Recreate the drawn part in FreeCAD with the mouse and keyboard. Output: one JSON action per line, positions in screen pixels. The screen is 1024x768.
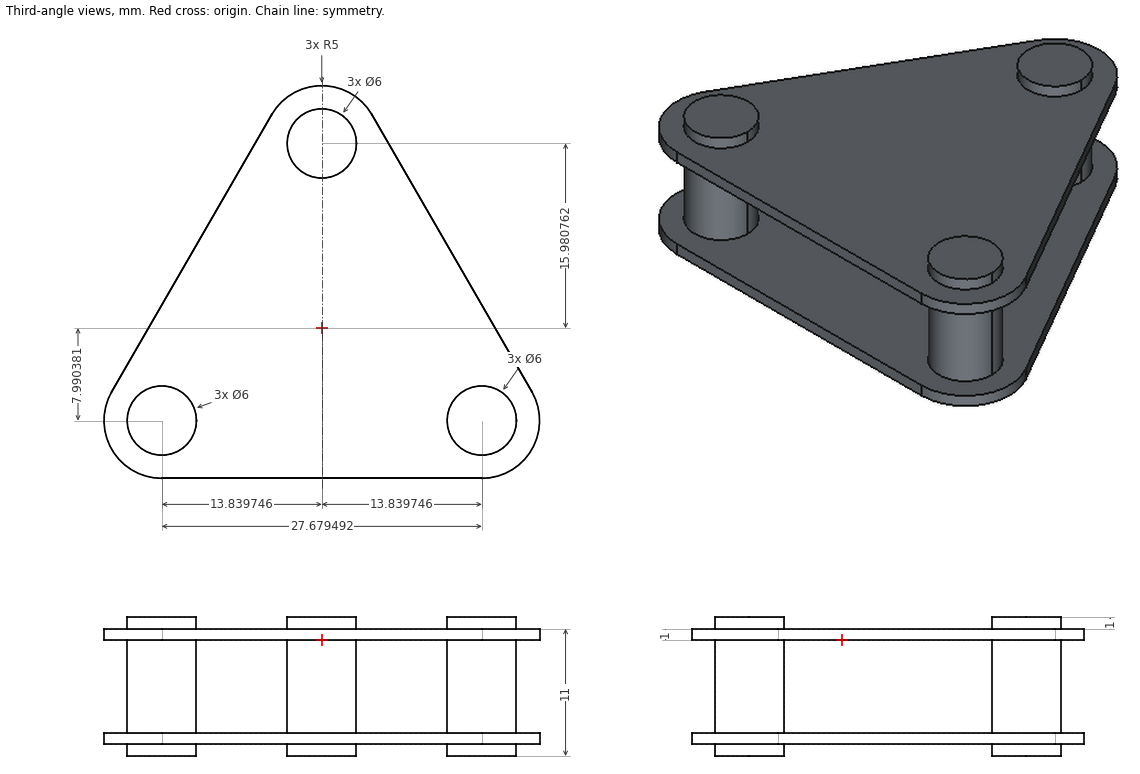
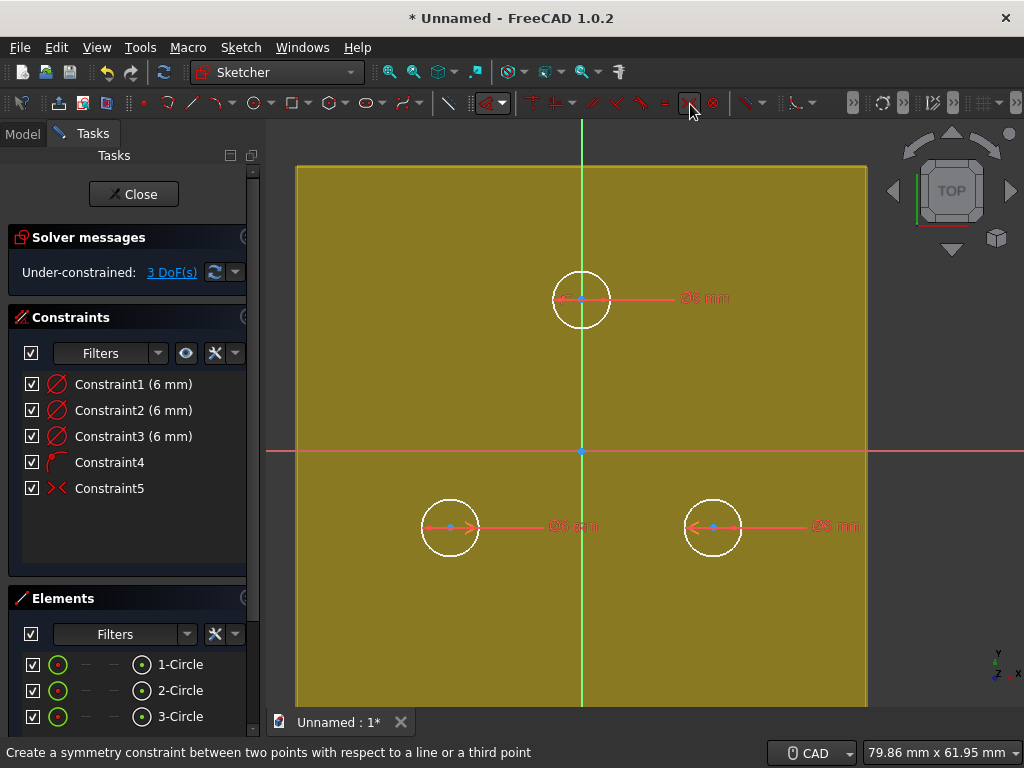
{"action": "left_click", "coordinate": [713, 528]}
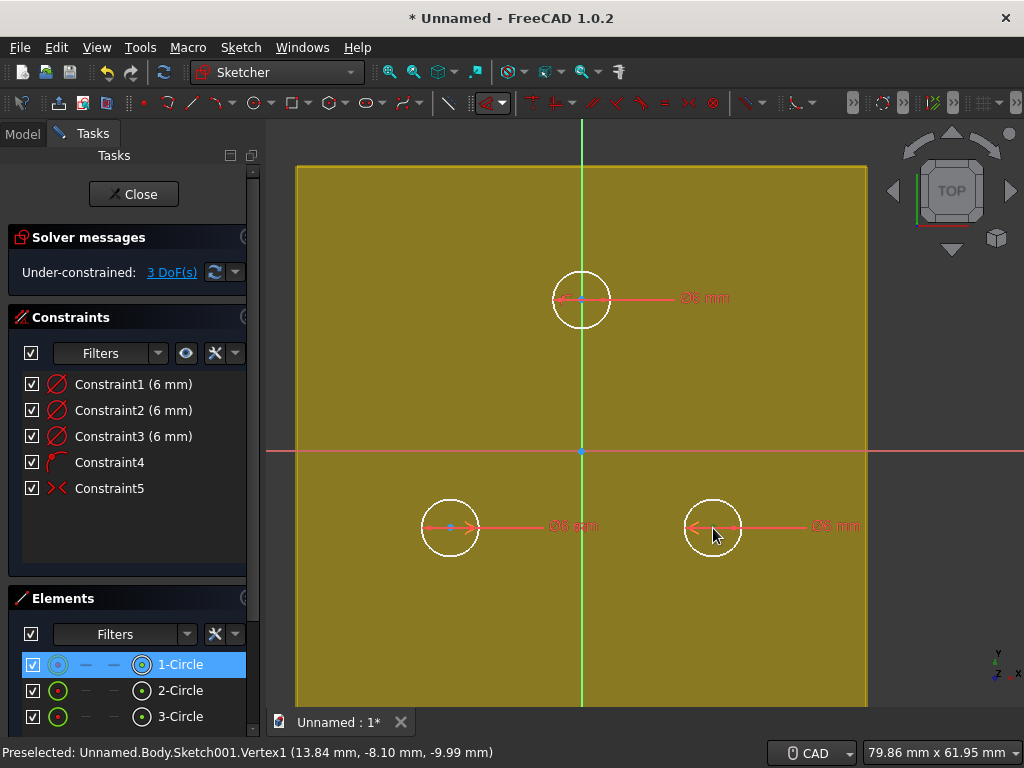
{"action": "left_click", "coordinate": [504, 104]}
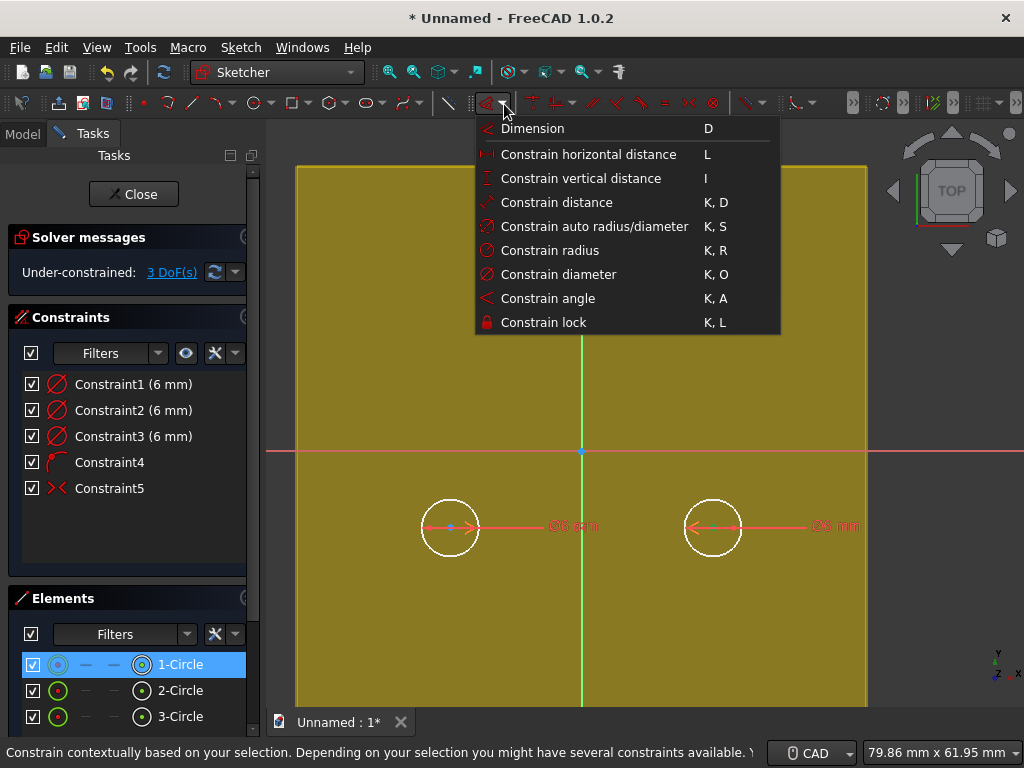
{"action": "left_click", "coordinate": [628, 178]}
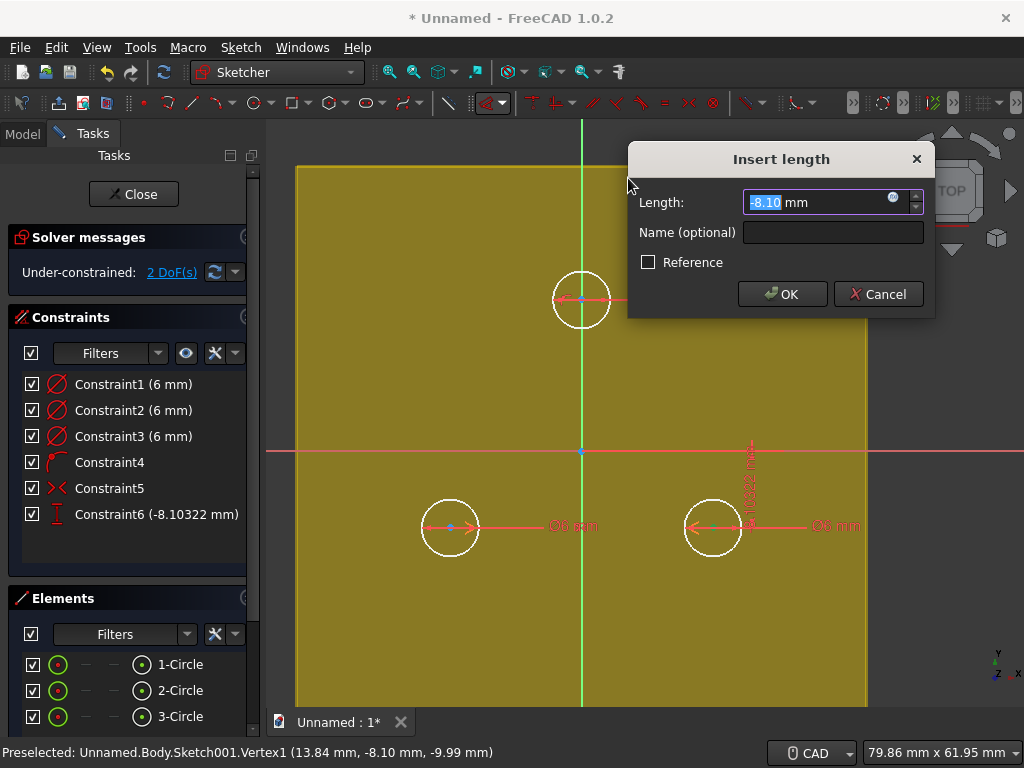
{"action": "type", "text": "-7.990381"}
{"action": "key", "text": "Return"}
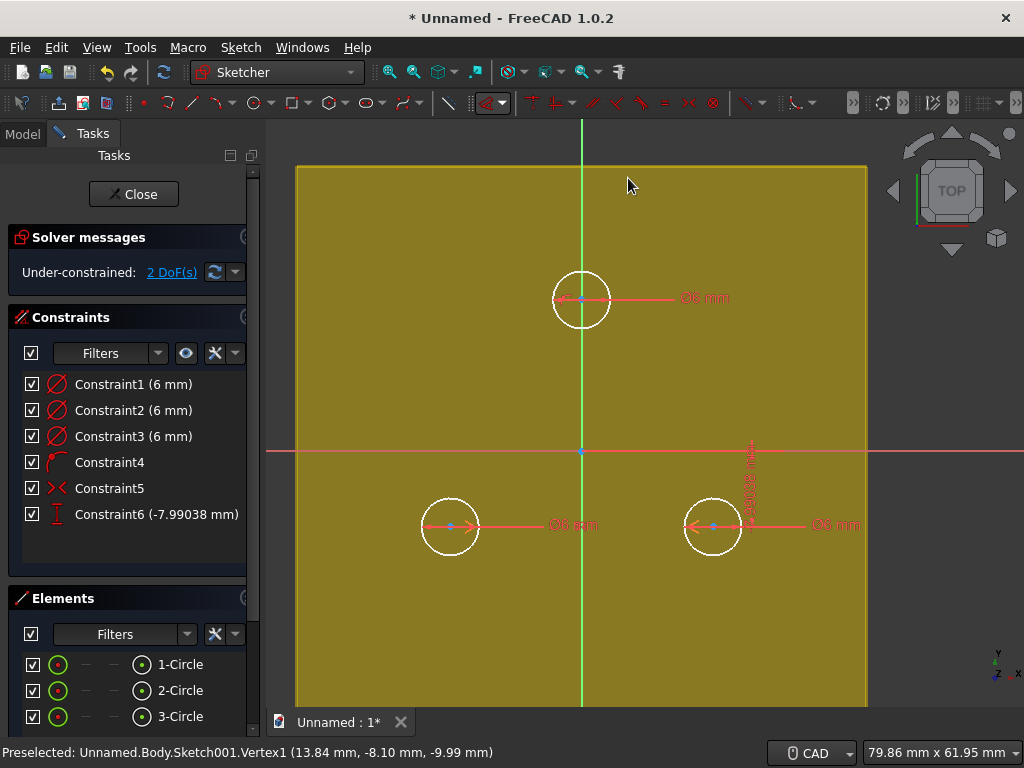
{"action": "left_click", "coordinate": [713, 527]}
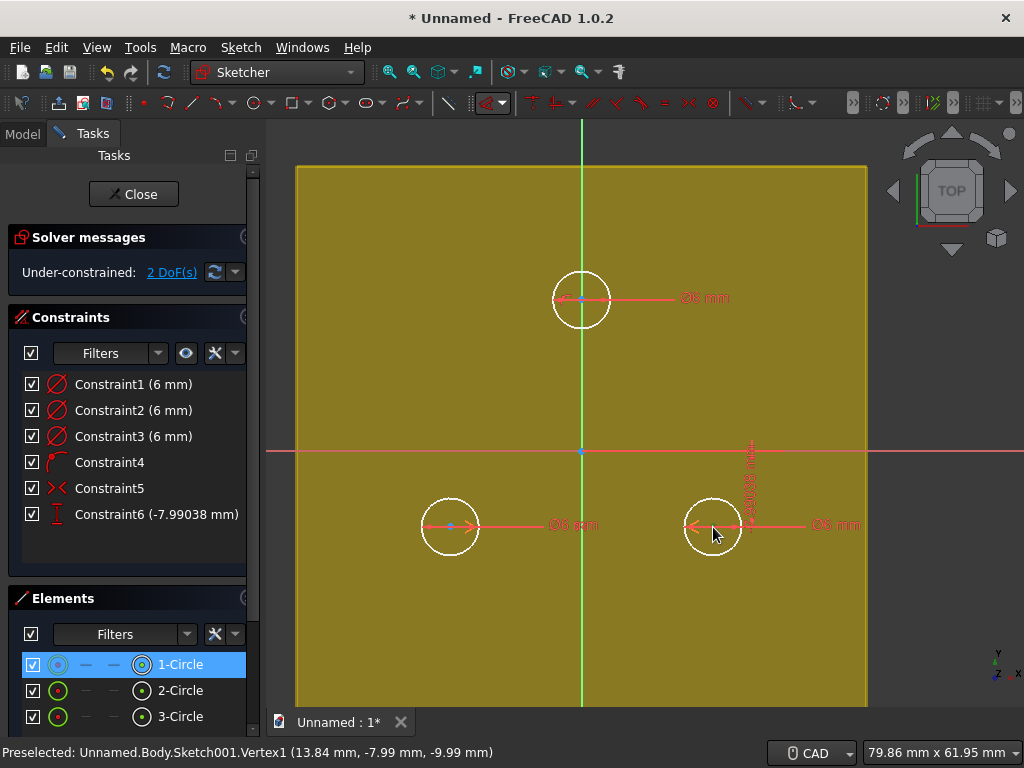
{"action": "key", "text": "l"}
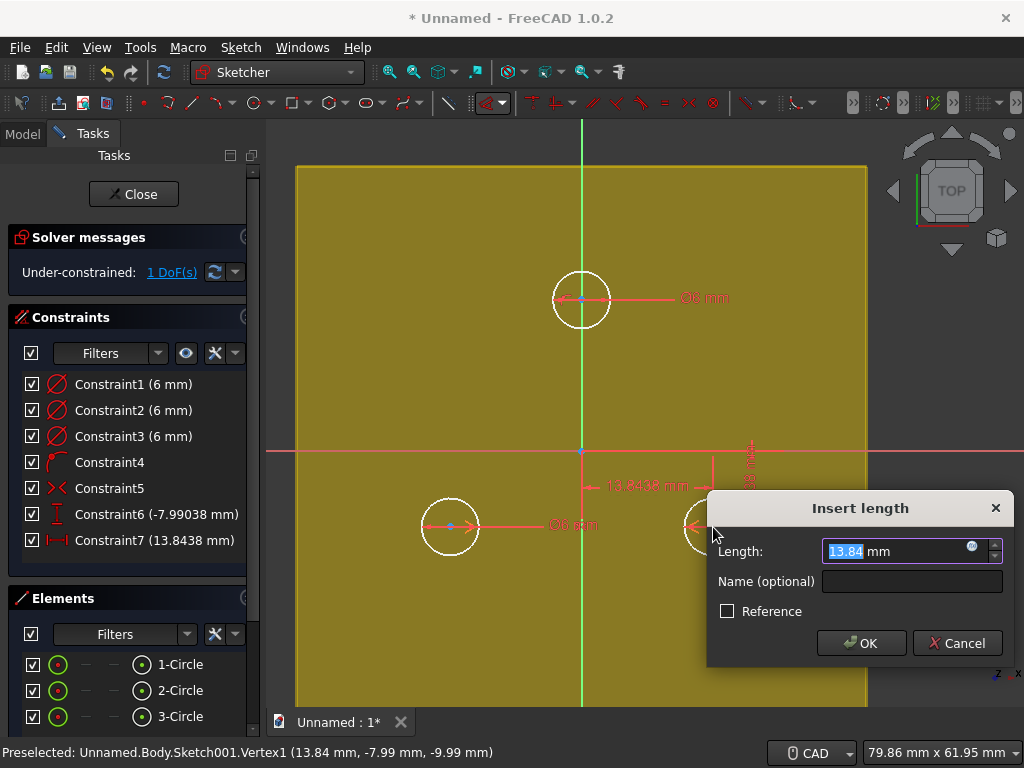
{"action": "type", "text": "13.839746"}
{"action": "key", "text": "Return"}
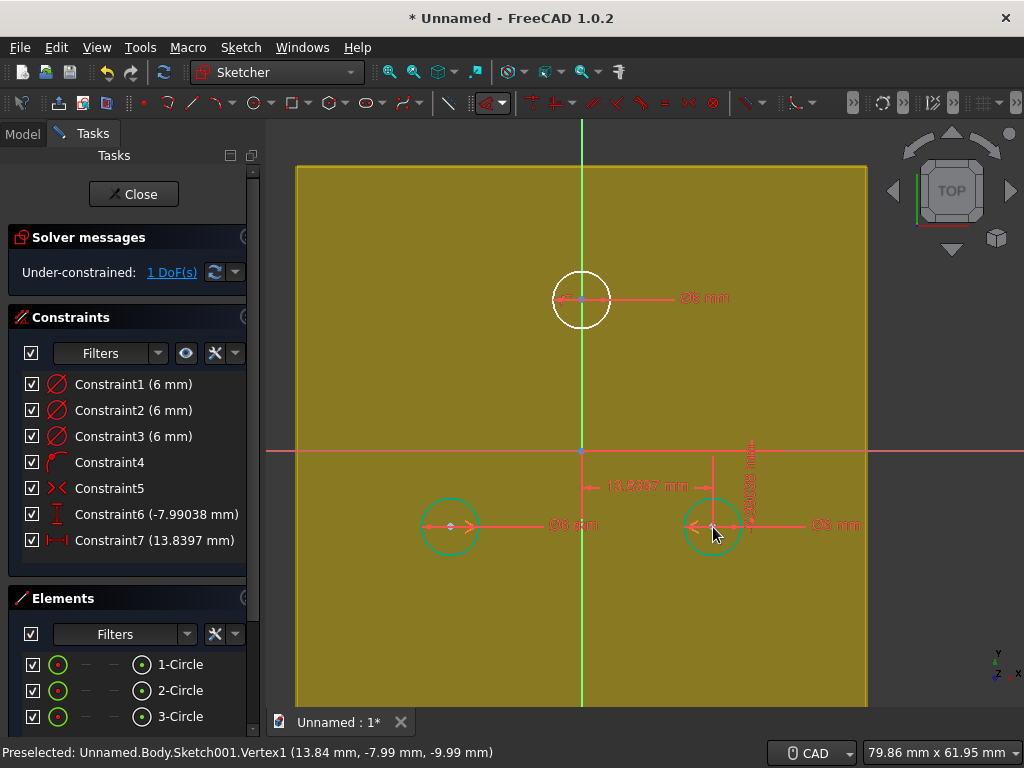
{"action": "left_click", "coordinate": [582, 300]}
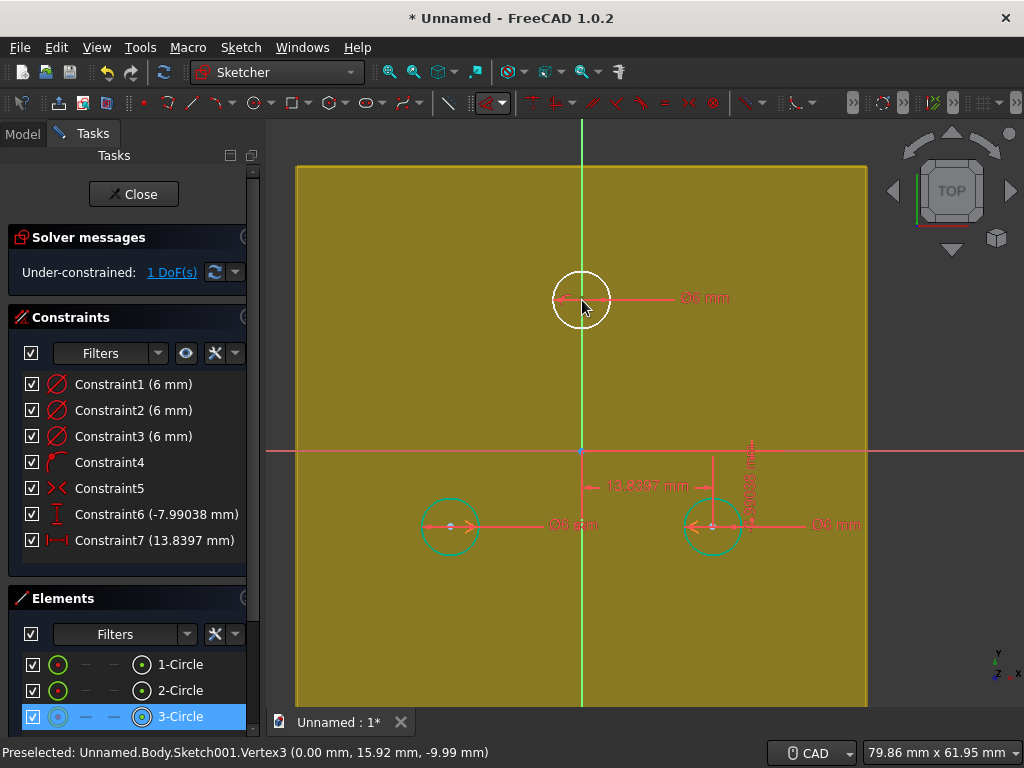
{"action": "key", "text": "i"}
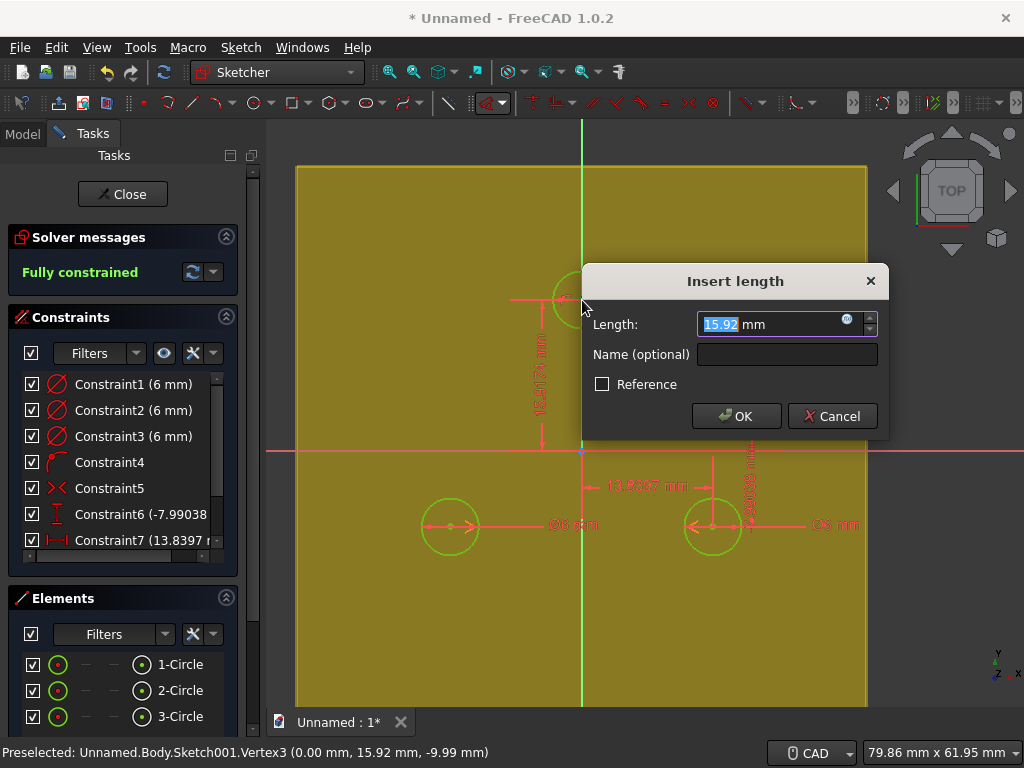
{"action": "type", "text": "15.980762"}
{"action": "key", "text": "Return"}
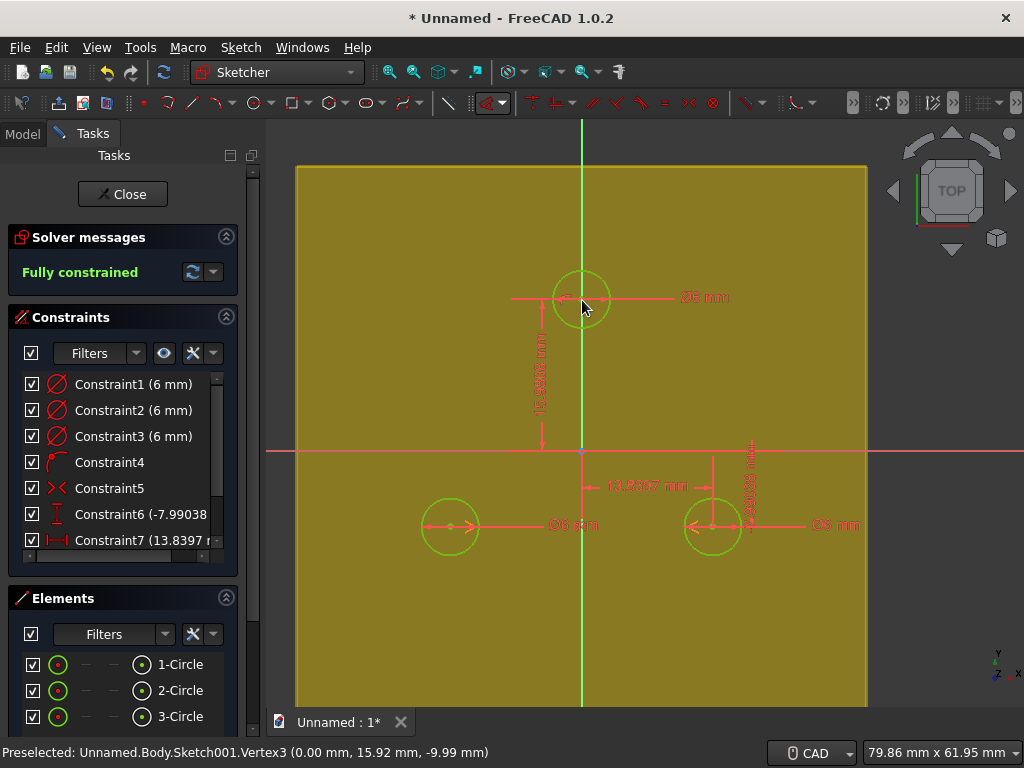
{"action": "left_click", "coordinate": [123, 194]}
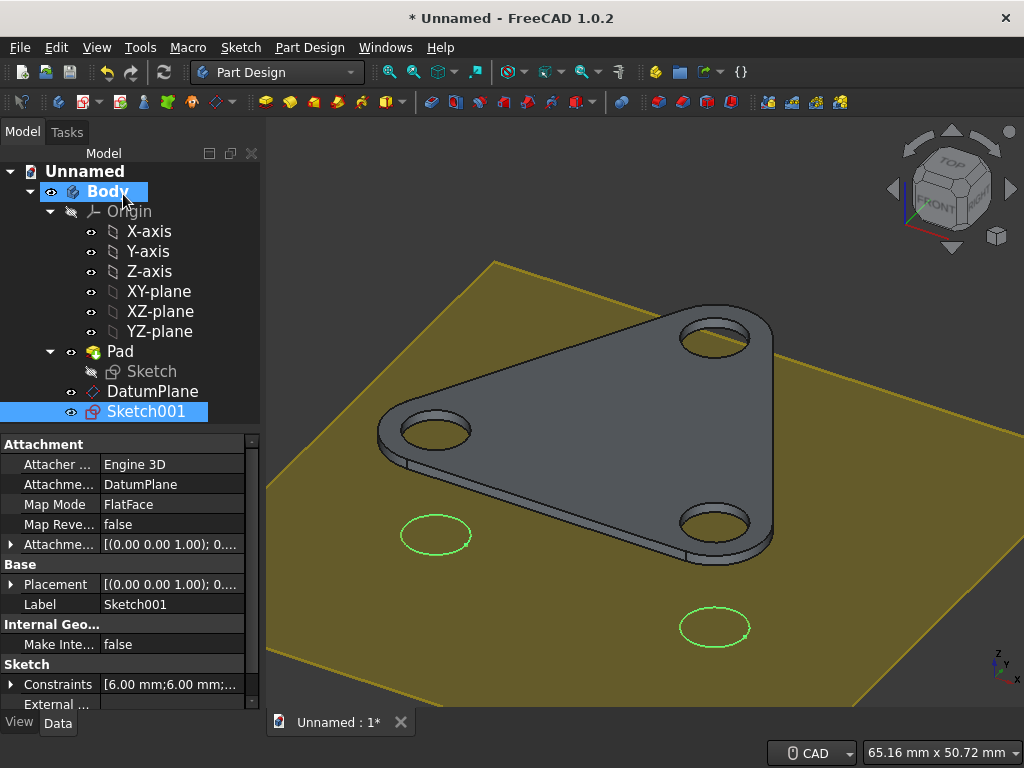
{"action": "left_click", "coordinate": [266, 102]}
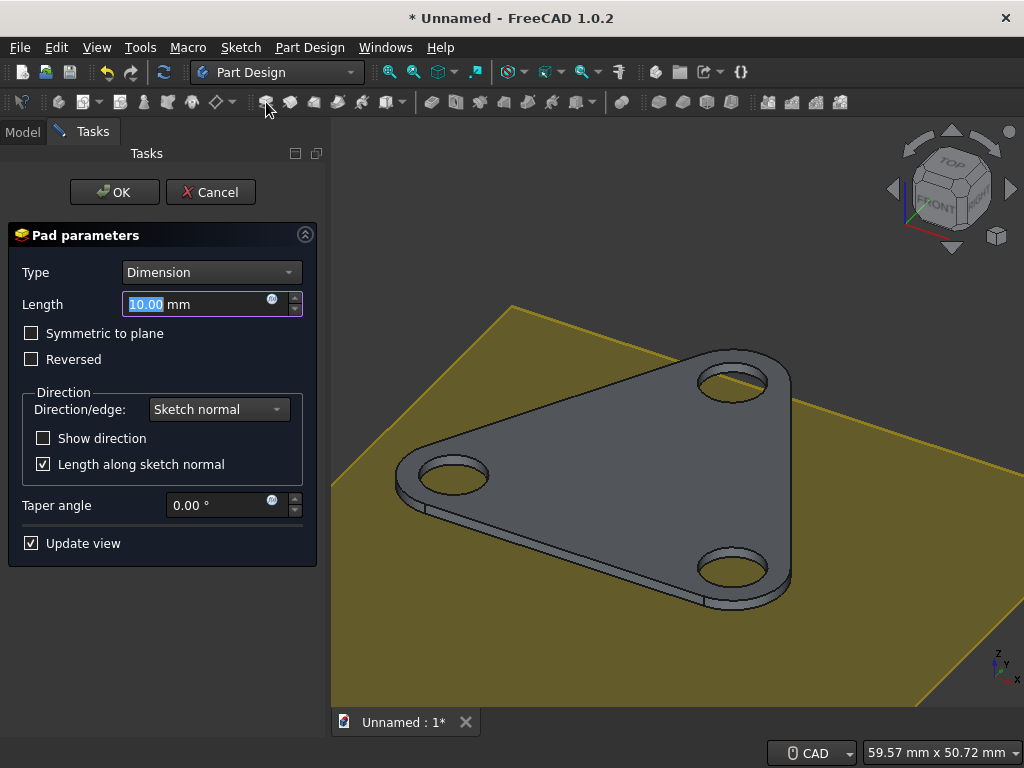
{"action": "type", "text": "11"}
{"action": "key", "text": "Tab"}